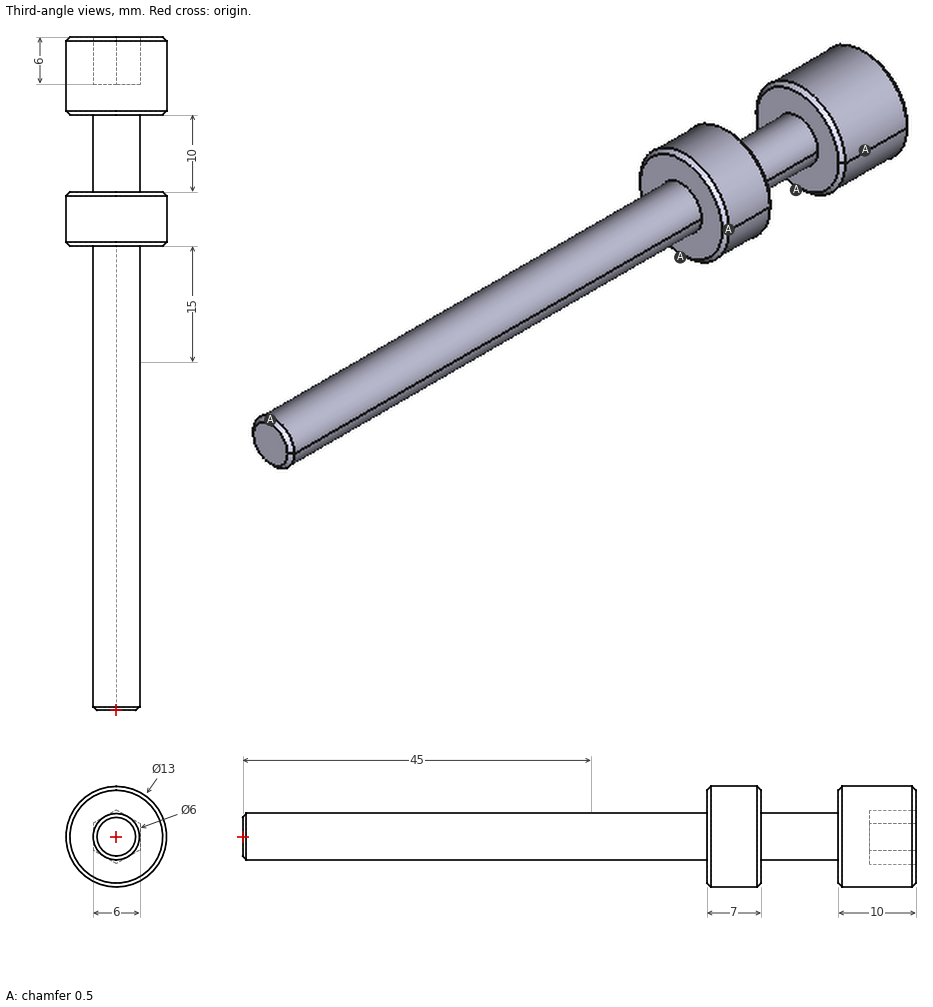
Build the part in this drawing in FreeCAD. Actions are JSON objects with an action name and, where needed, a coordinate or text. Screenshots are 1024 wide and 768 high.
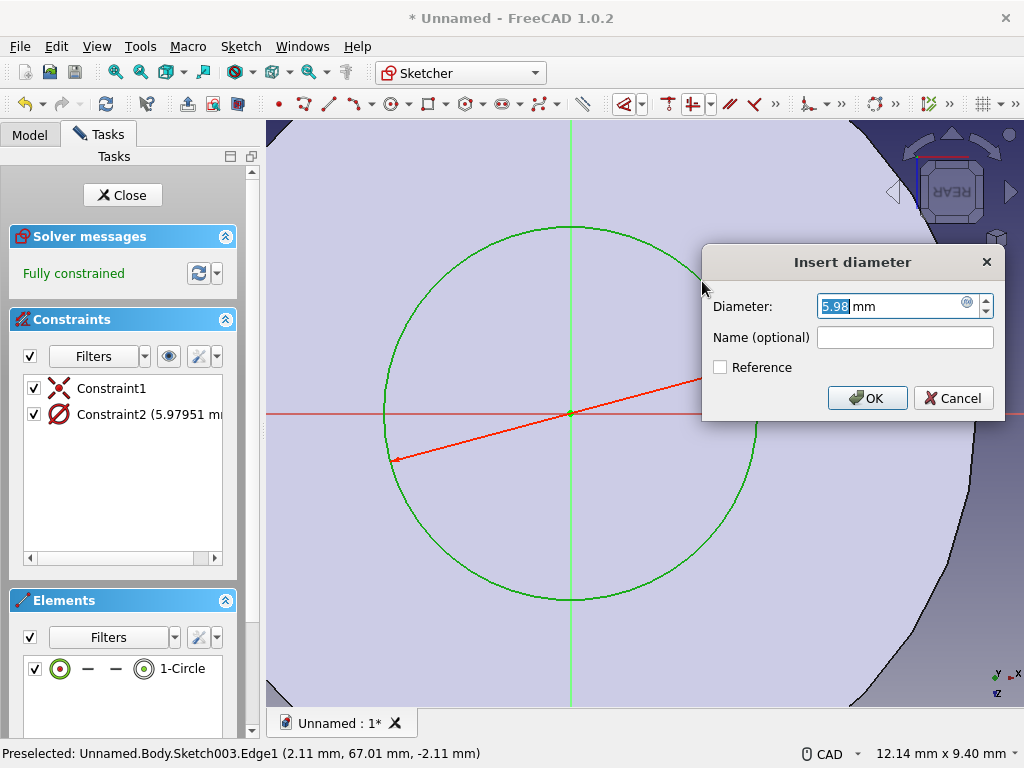
{"action": "type", "text": "6"}
{"action": "key", "text": "Return"}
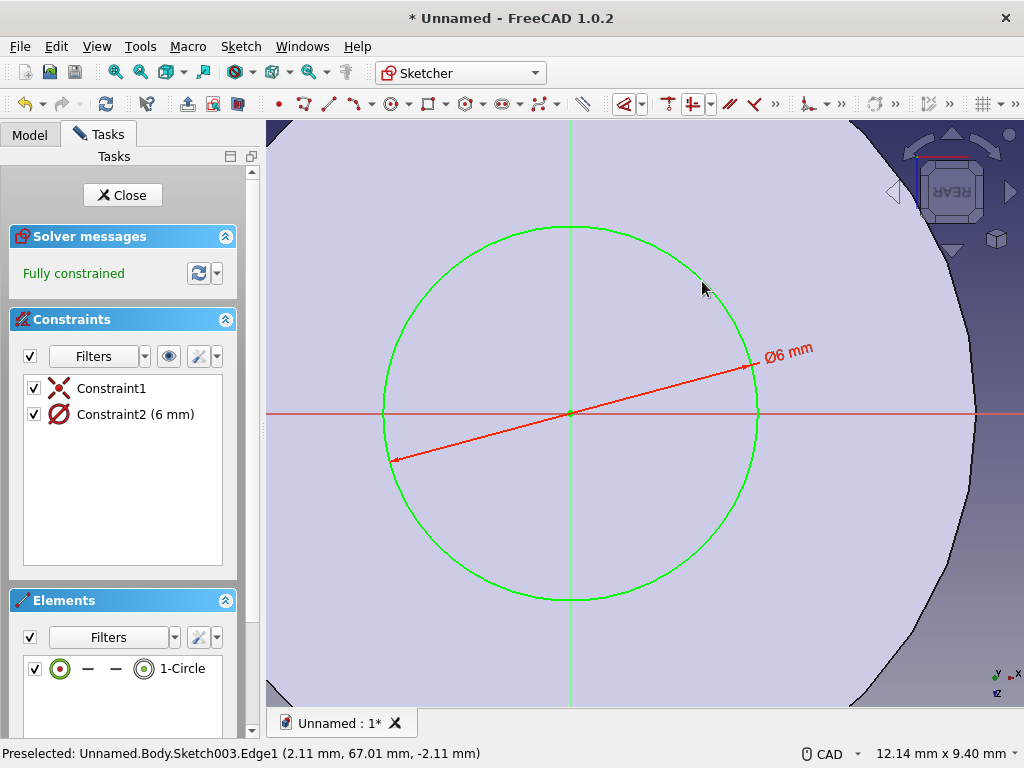
{"action": "left_click", "coordinate": [123, 195]}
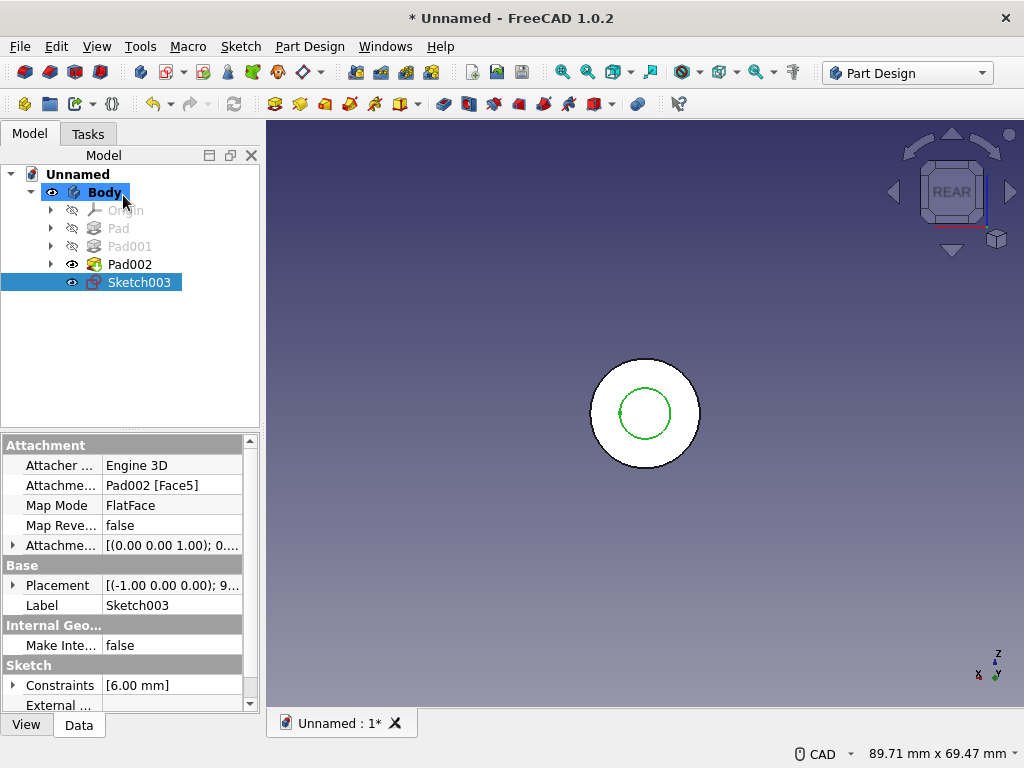
{"action": "left_click", "coordinate": [275, 104]}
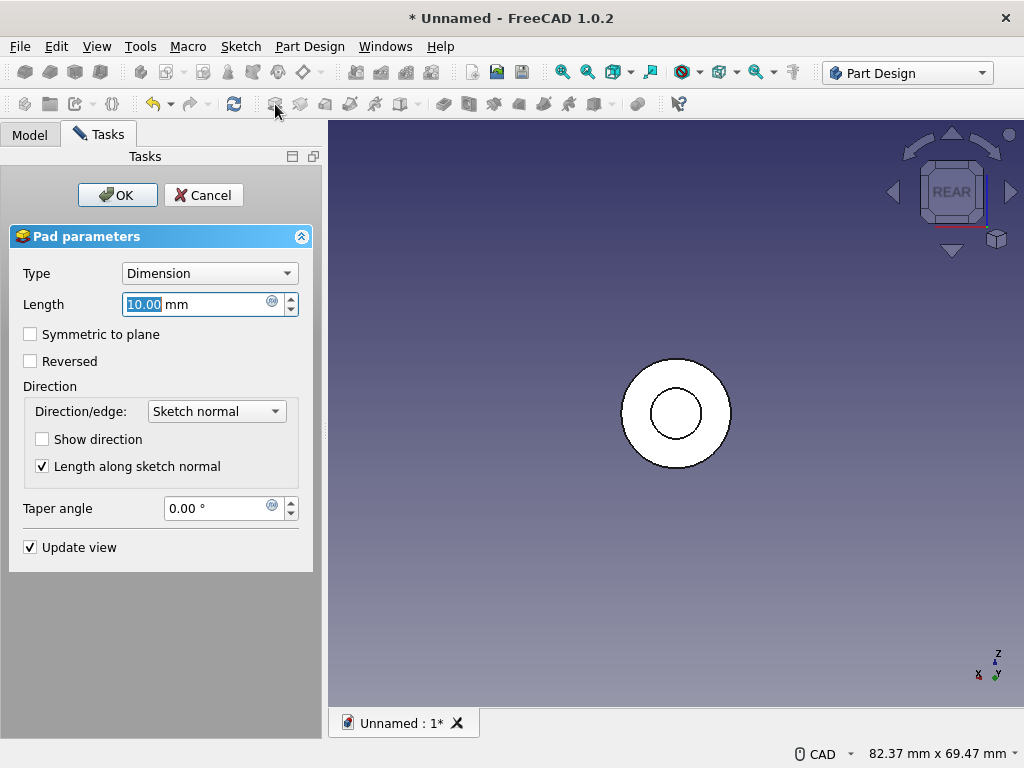
{"action": "type", "text": "10"}
{"action": "key", "text": "Tab"}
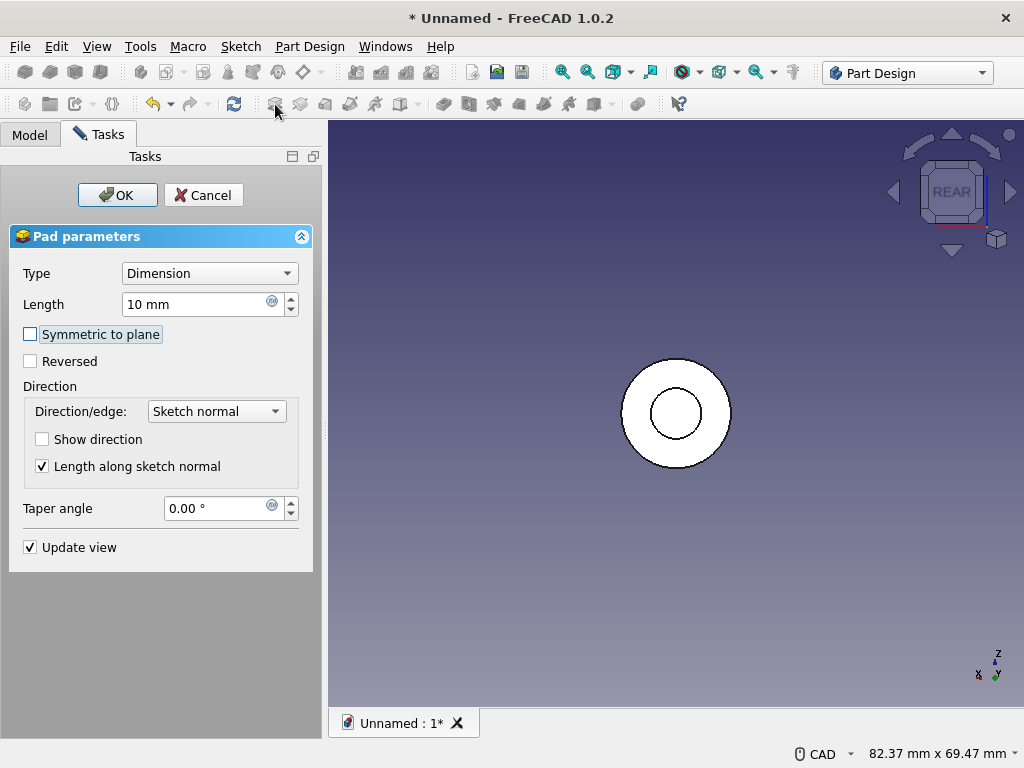
{"action": "left_click", "coordinate": [118, 195]}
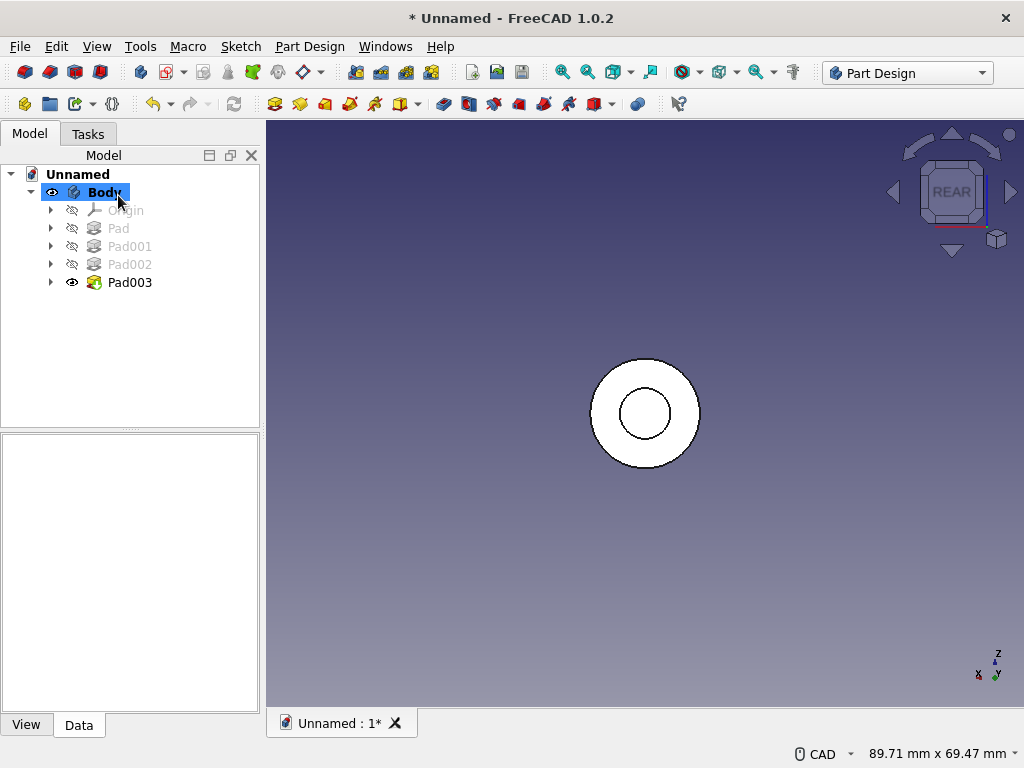
{"action": "left_click", "coordinate": [563, 72]}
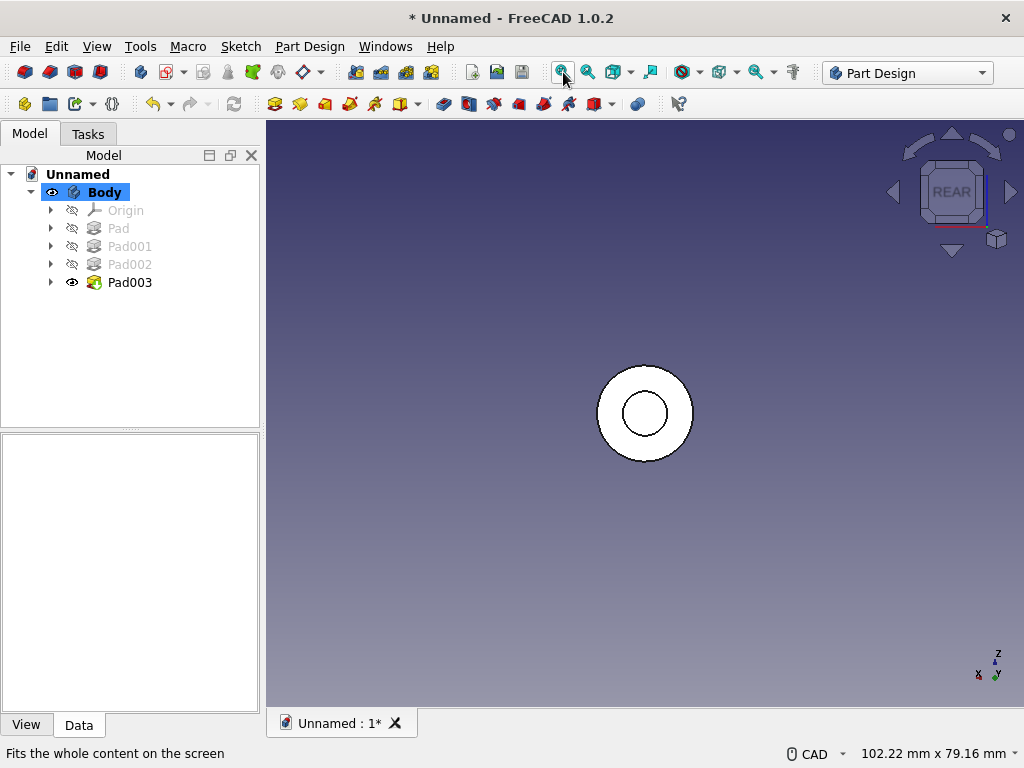
{"action": "left_click", "coordinate": [645, 412]}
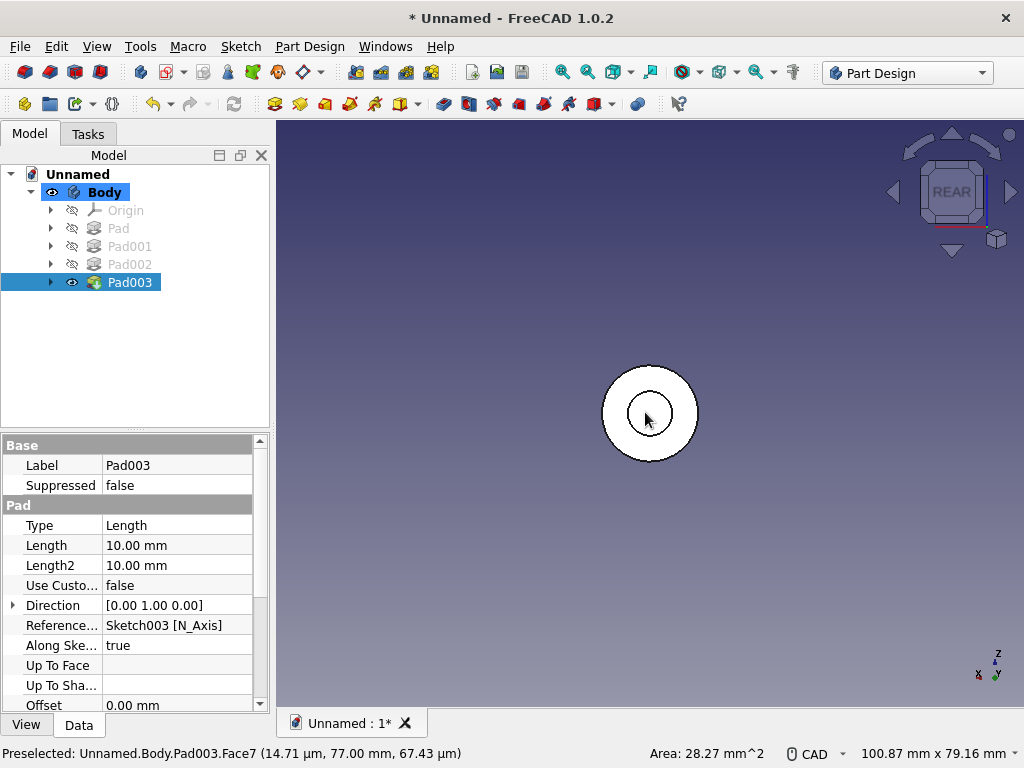
{"action": "left_click", "coordinate": [166, 72]}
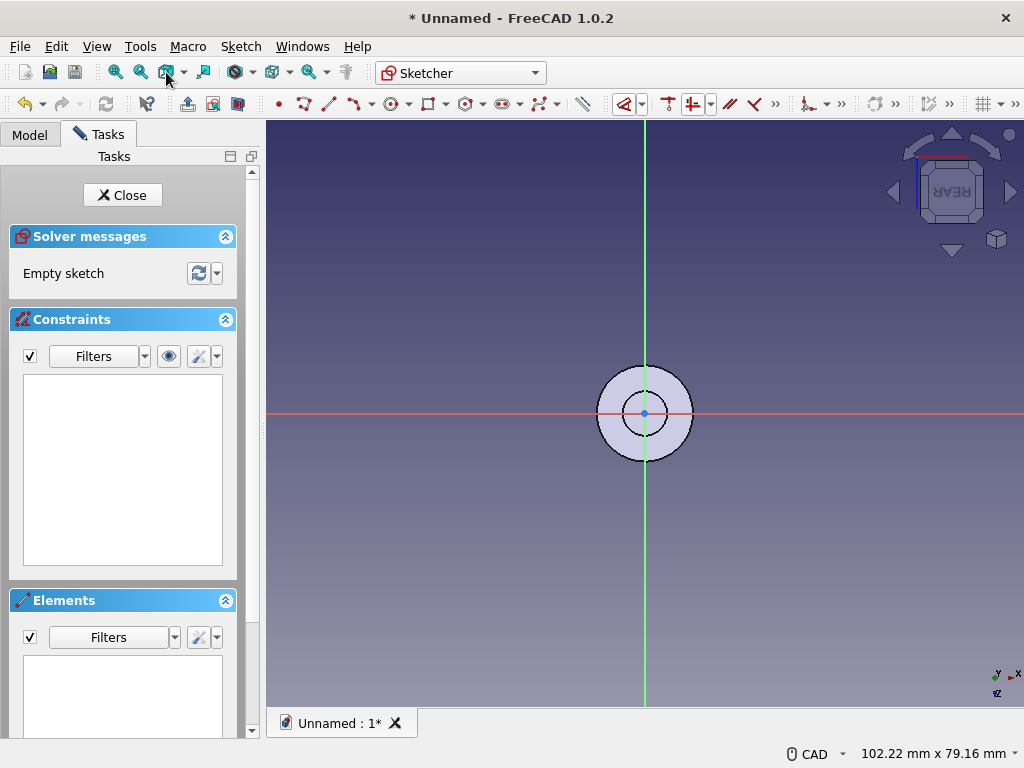
{"action": "scroll", "coordinate": [667, 413], "scroll_direction": "up", "scroll_amount": 7}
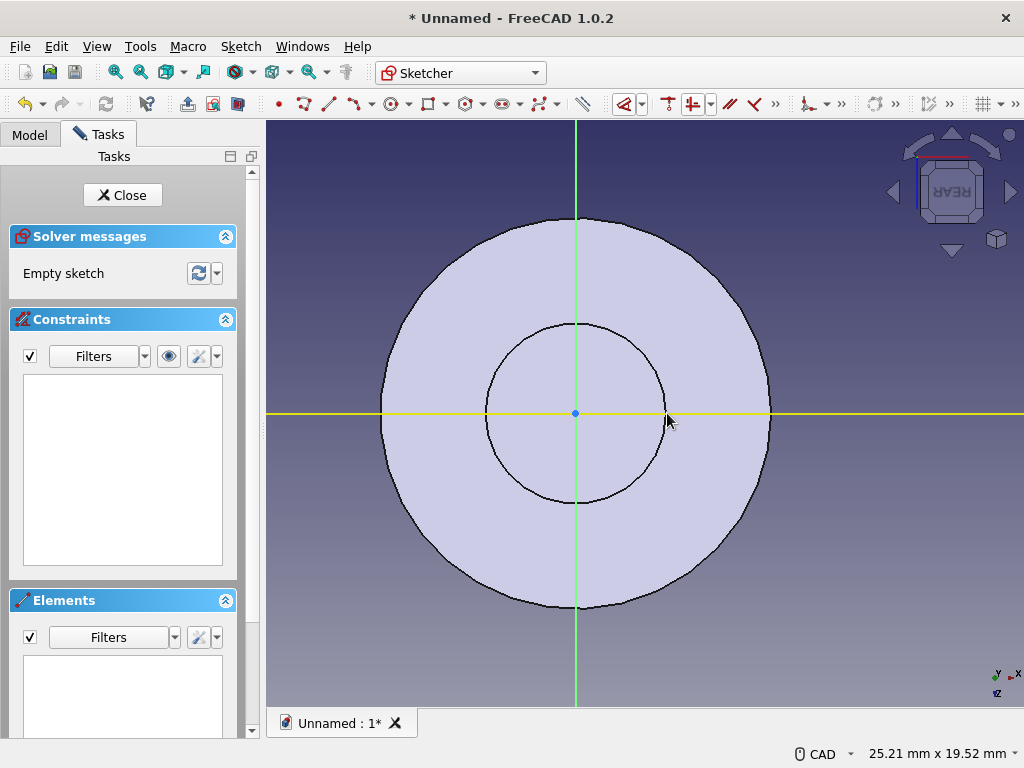
{"action": "left_click", "coordinate": [390, 104]}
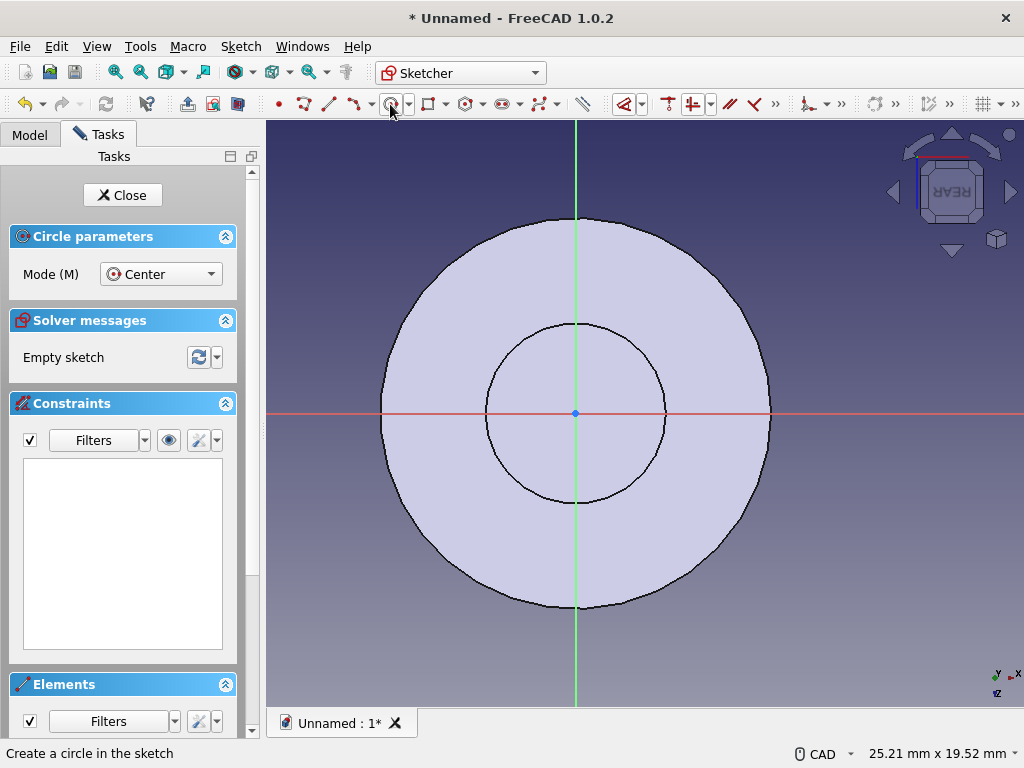
{"action": "left_click", "coordinate": [576, 413]}
{"action": "left_click", "coordinate": [714, 275]}
{"action": "key", "text": "Escape"}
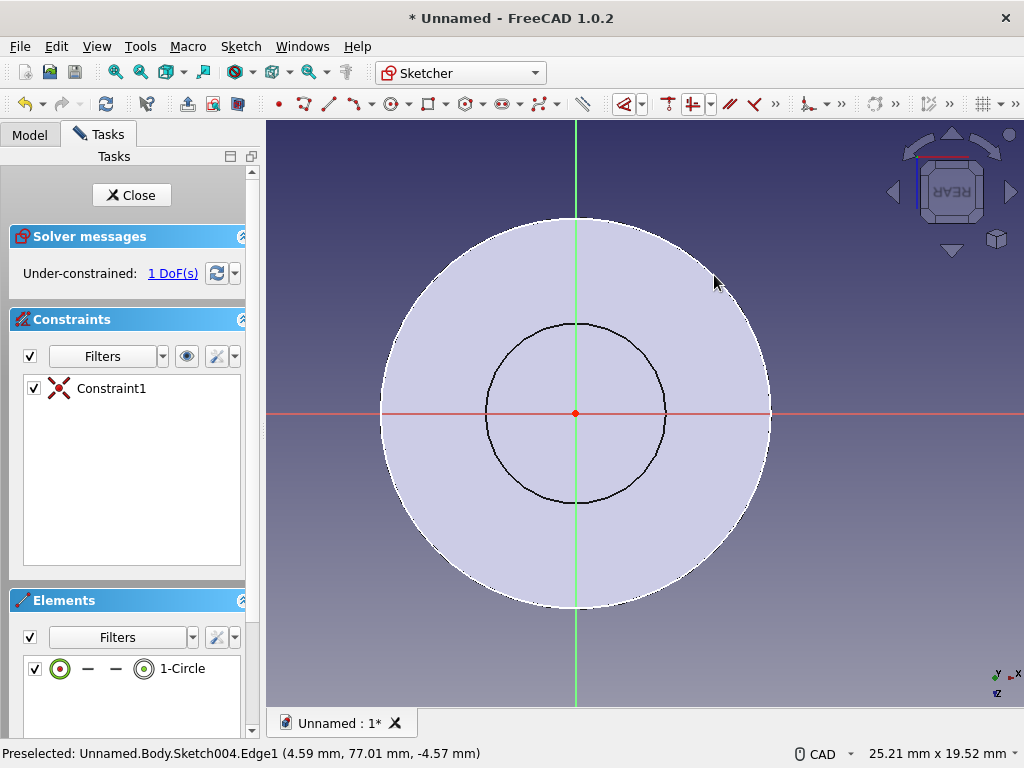
{"action": "left_click", "coordinate": [713, 275]}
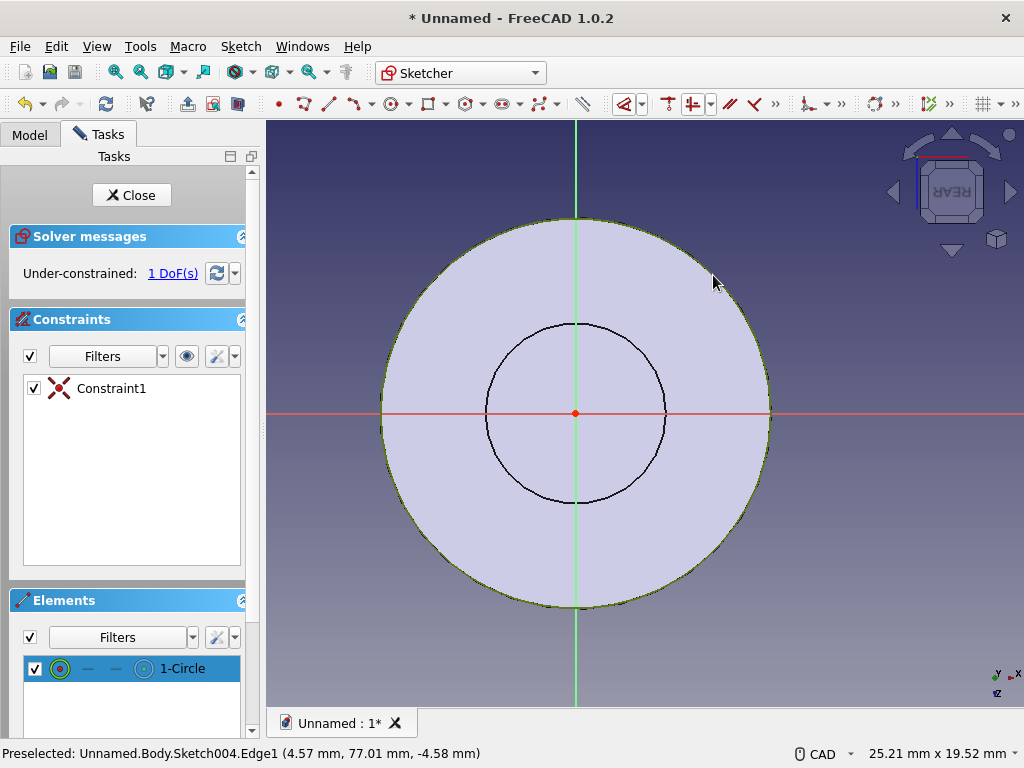
{"action": "key", "text": "k o"}